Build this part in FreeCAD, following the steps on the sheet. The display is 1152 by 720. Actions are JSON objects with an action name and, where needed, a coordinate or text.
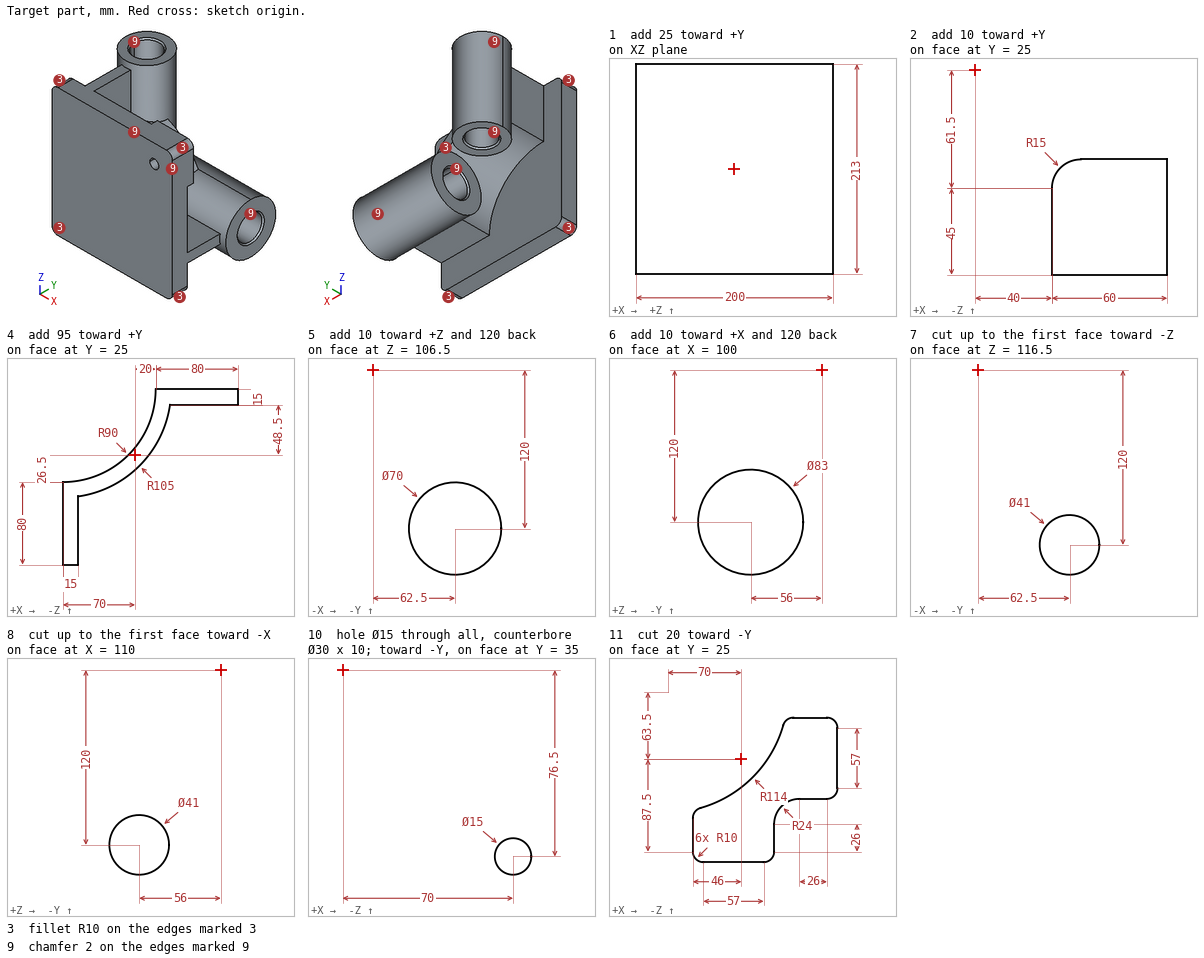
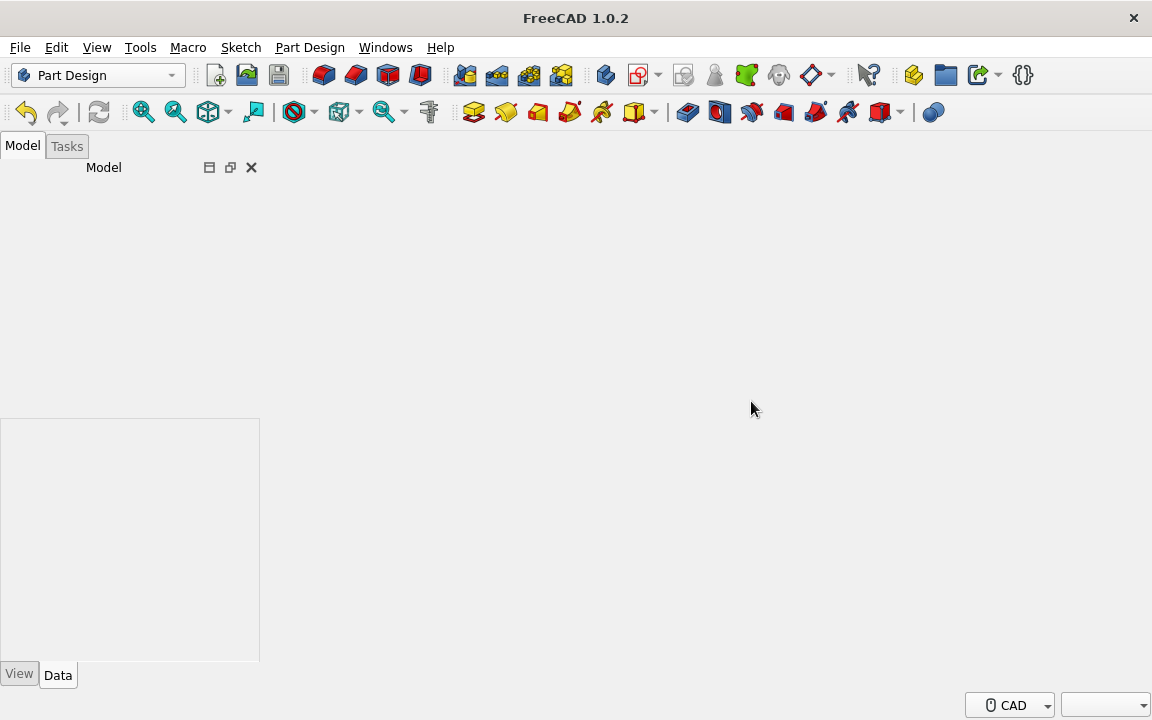
{"action": "left_click", "coordinate": [216, 76]}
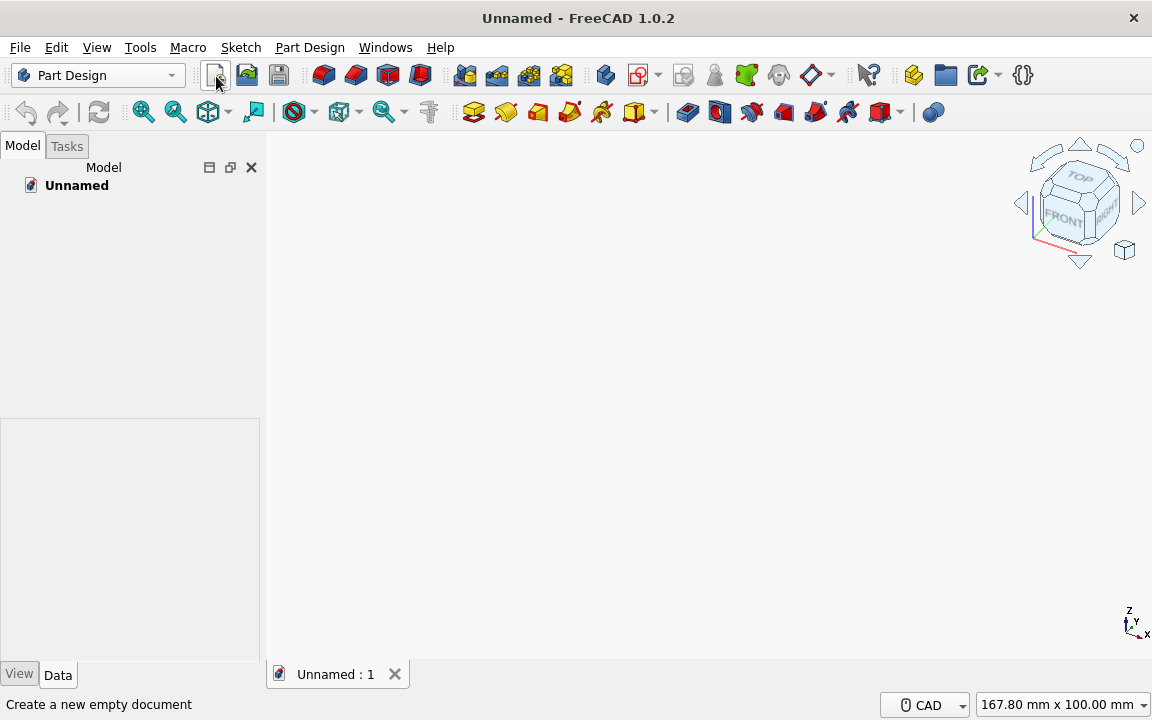
{"action": "left_click", "coordinate": [638, 76]}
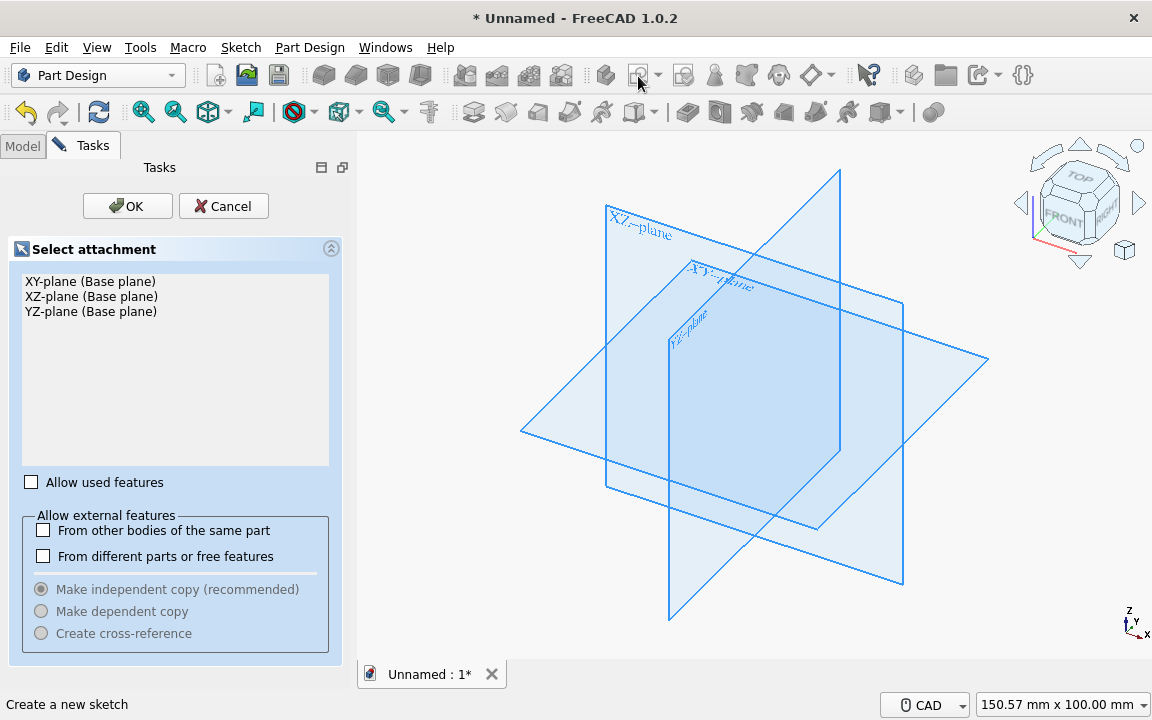
{"action": "left_click", "coordinate": [82, 296]}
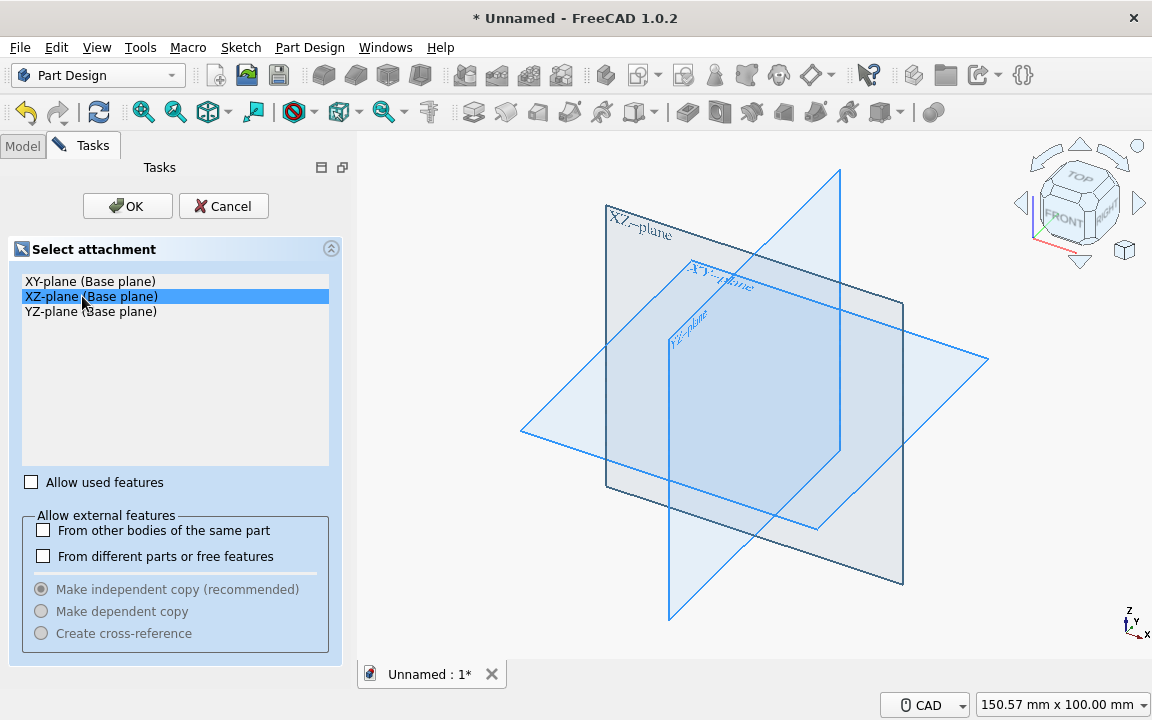
{"action": "left_click", "coordinate": [128, 206]}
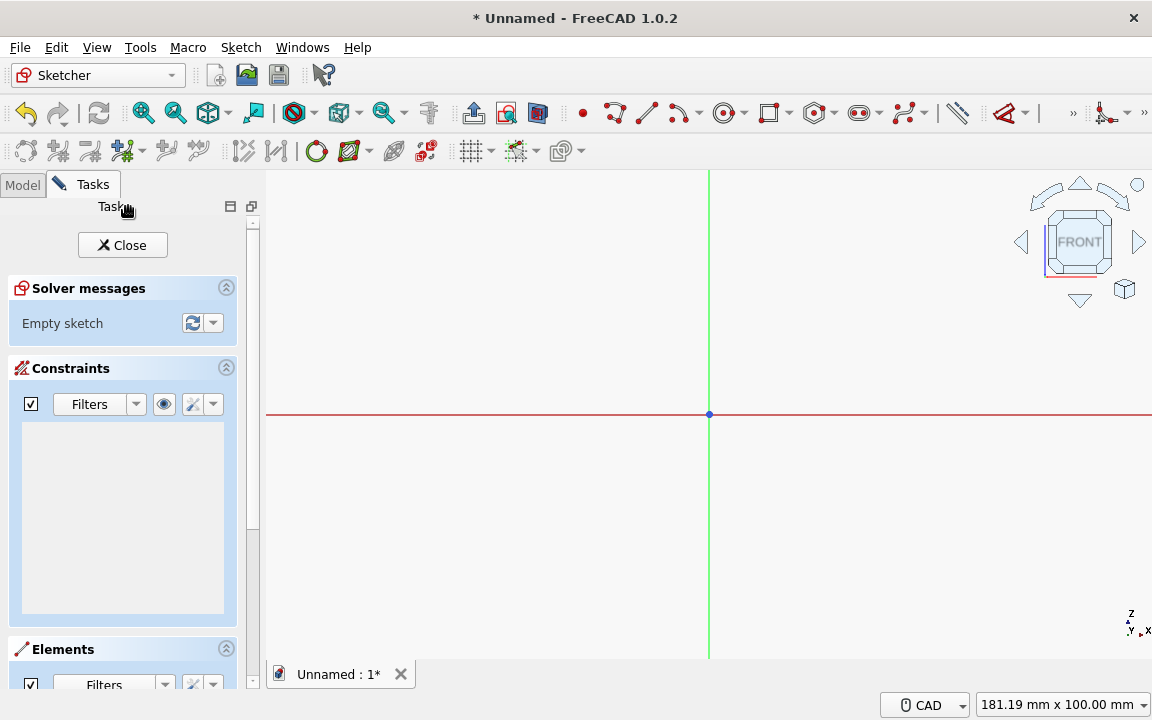
{"action": "scroll", "coordinate": [611, 414], "scroll_direction": "down", "scroll_amount": 6}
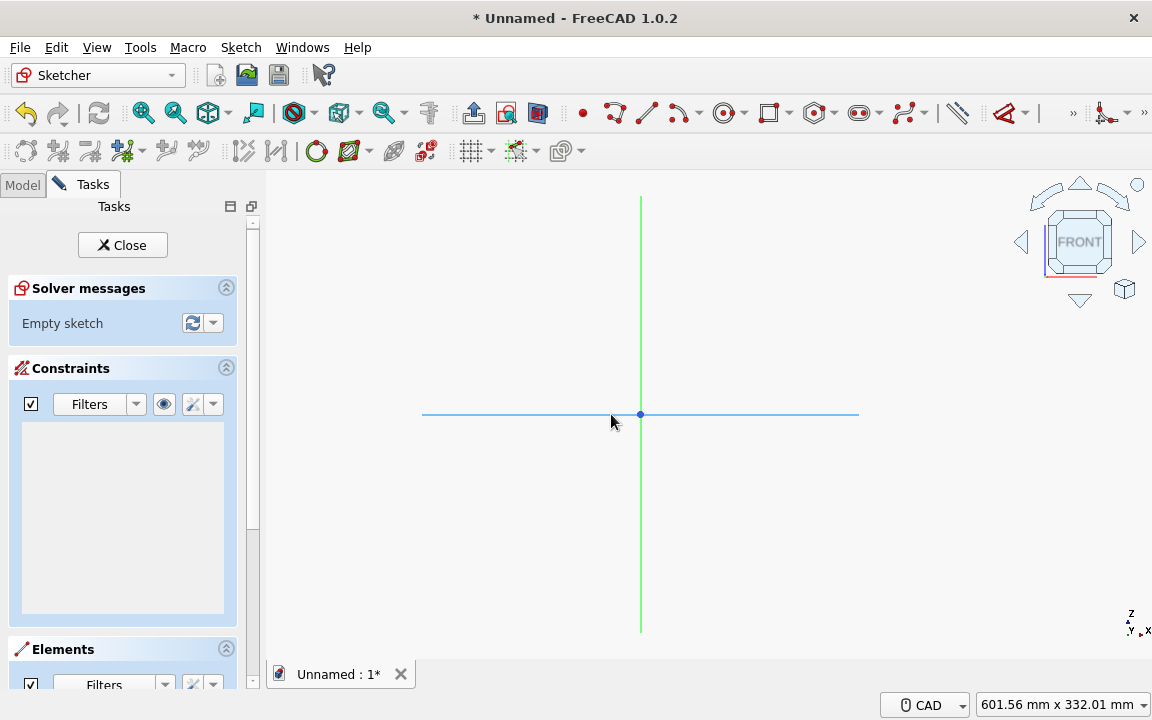
{"action": "left_click", "coordinate": [792, 114]}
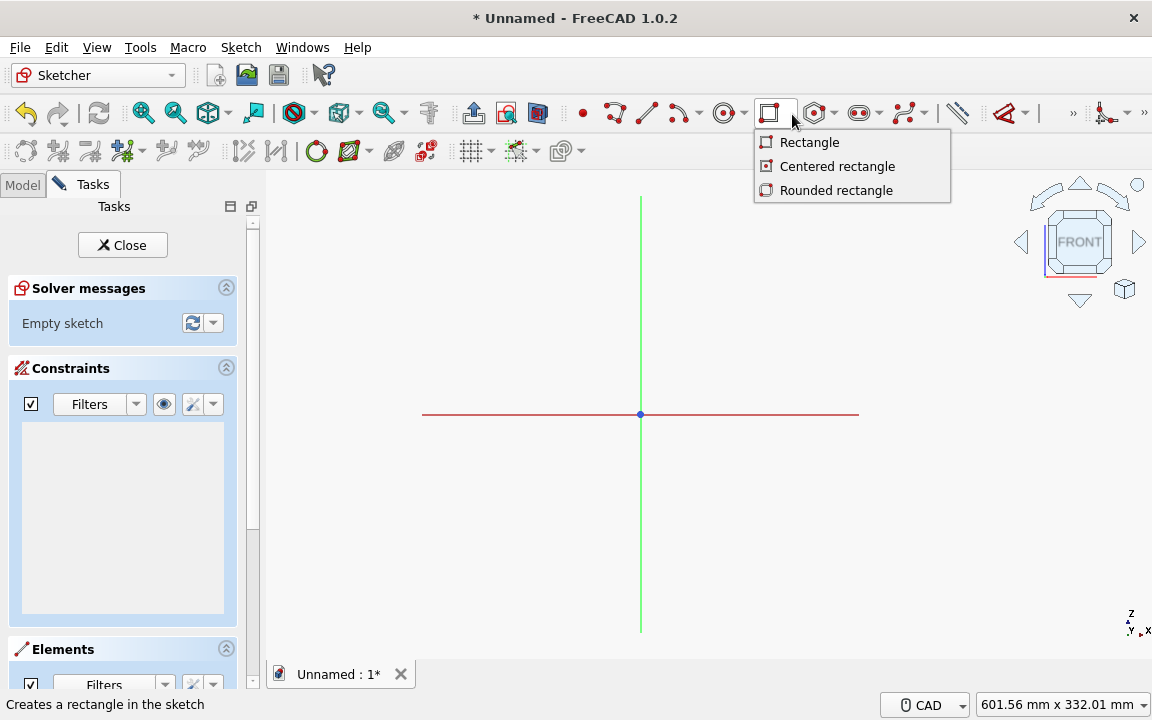
{"action": "left_click", "coordinate": [852, 166]}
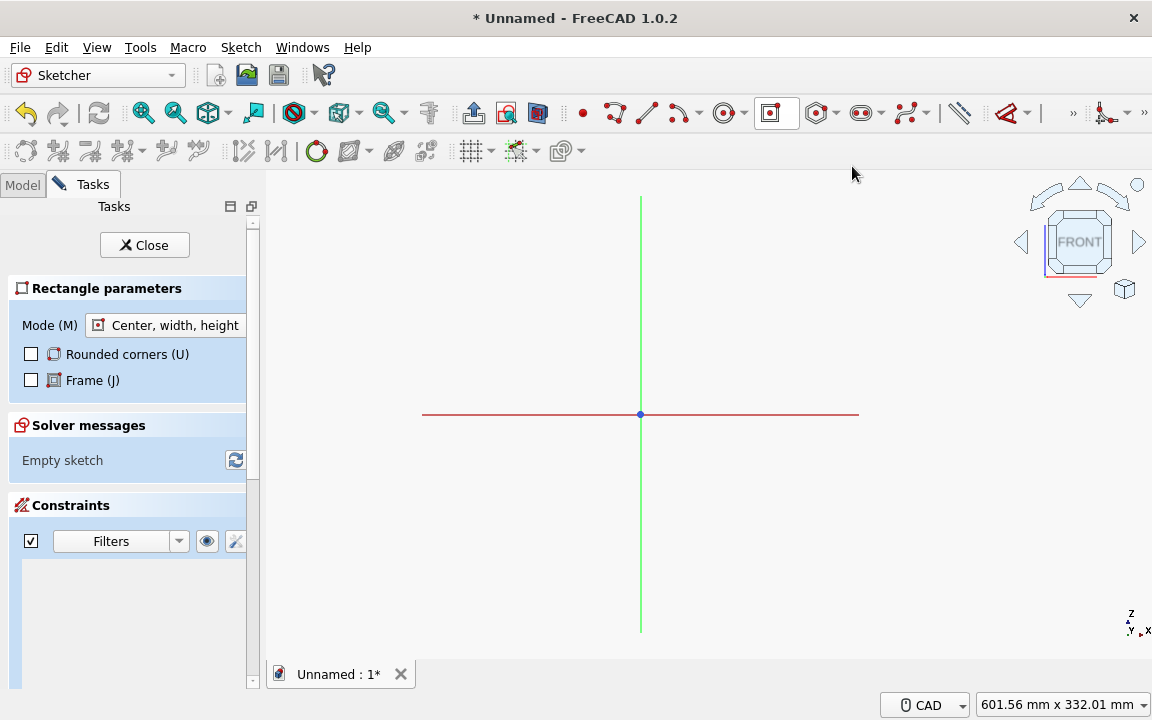
{"action": "left_click", "coordinate": [641, 414]}
{"action": "mouse_move", "coordinate": [788, 258]}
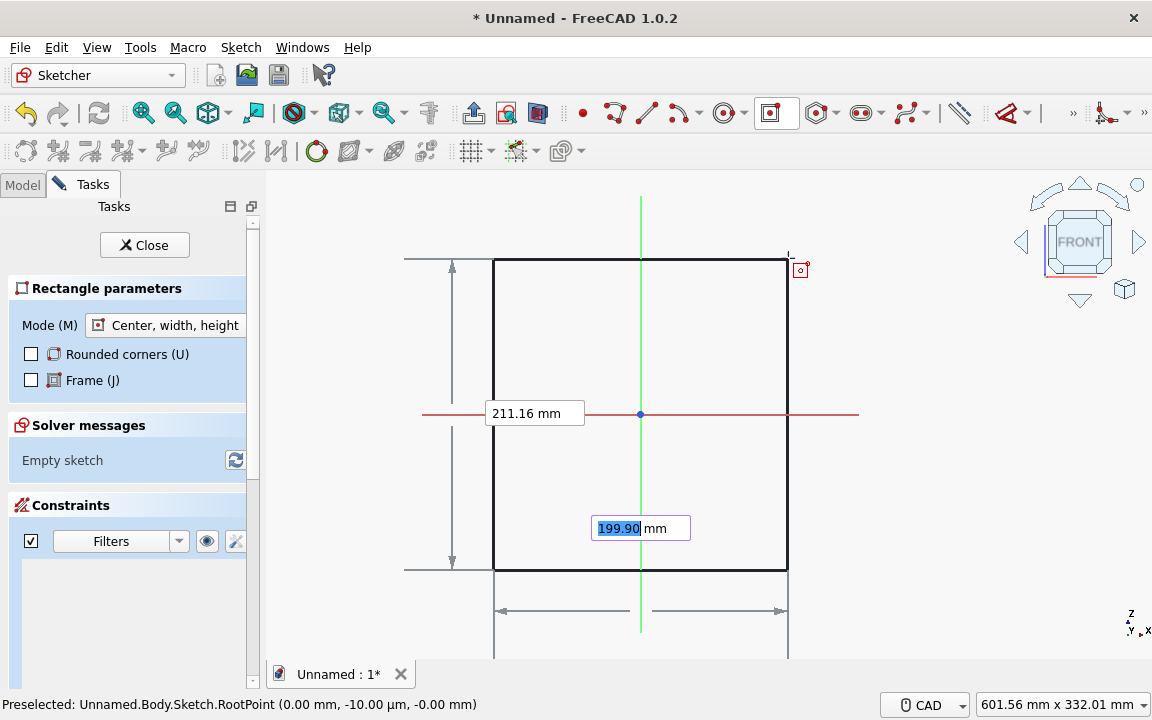
{"action": "type", "text": "200"}
{"action": "key", "text": "Tab"}
{"action": "type", "text": "213"}
{"action": "key", "text": "Return"}
{"action": "key", "text": "Escape"}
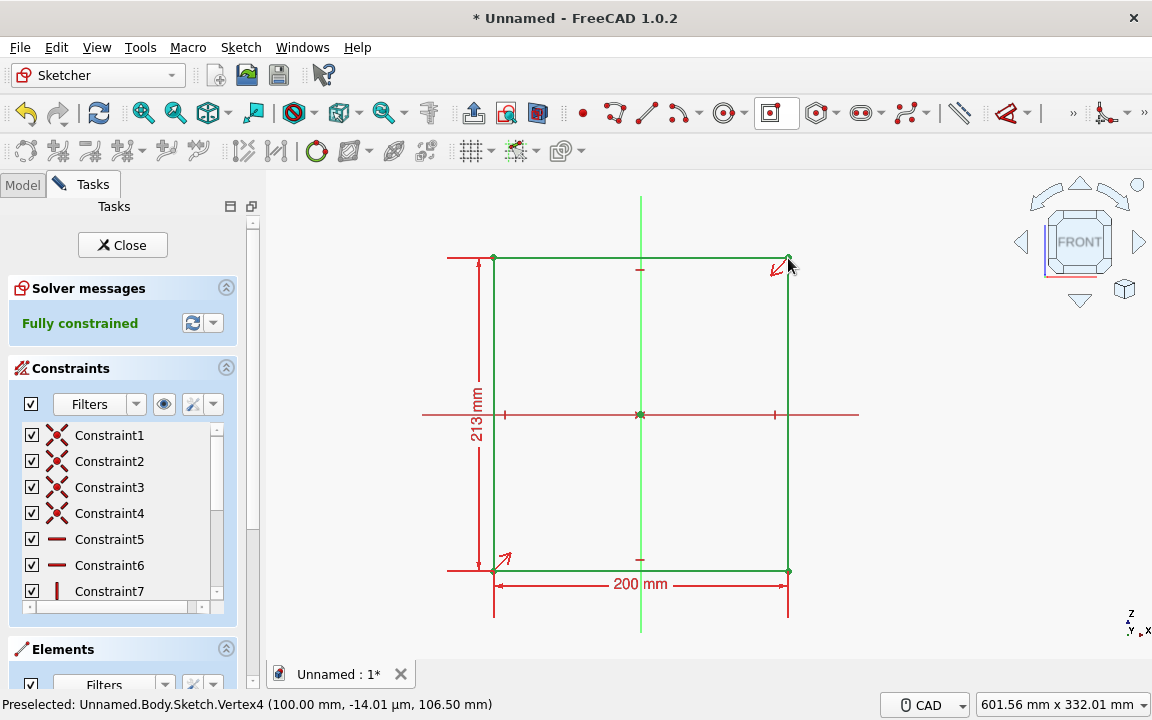
{"action": "left_click", "coordinate": [123, 245]}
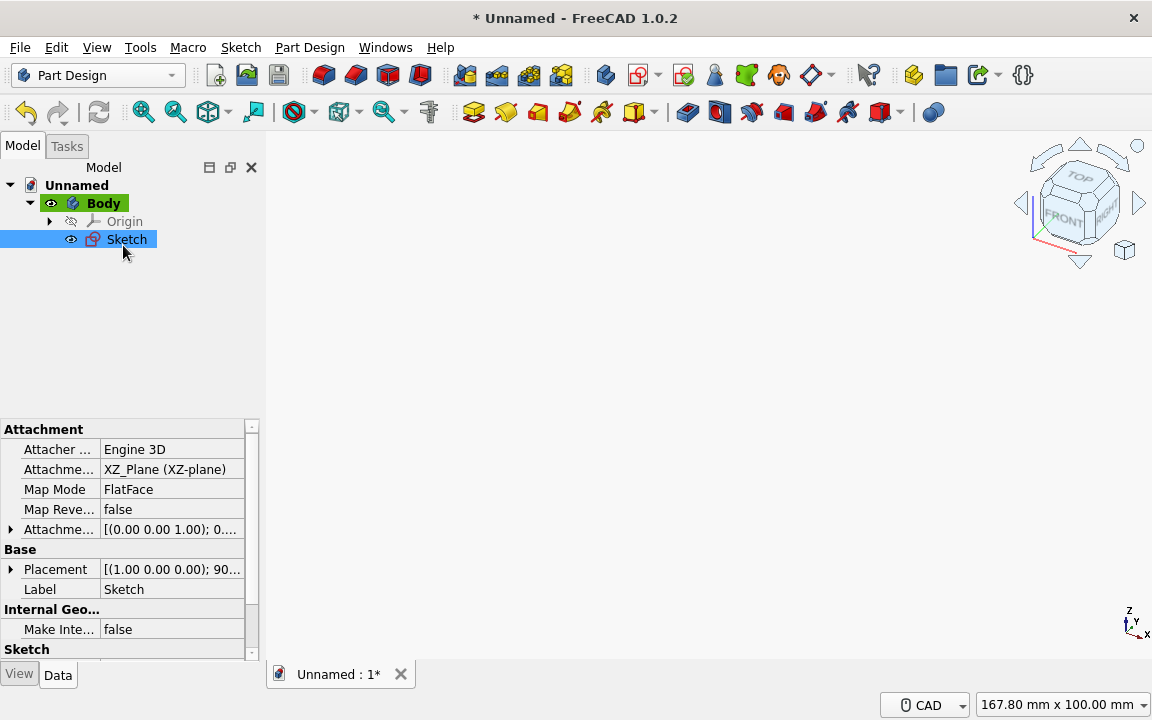
{"action": "left_click", "coordinate": [474, 112]}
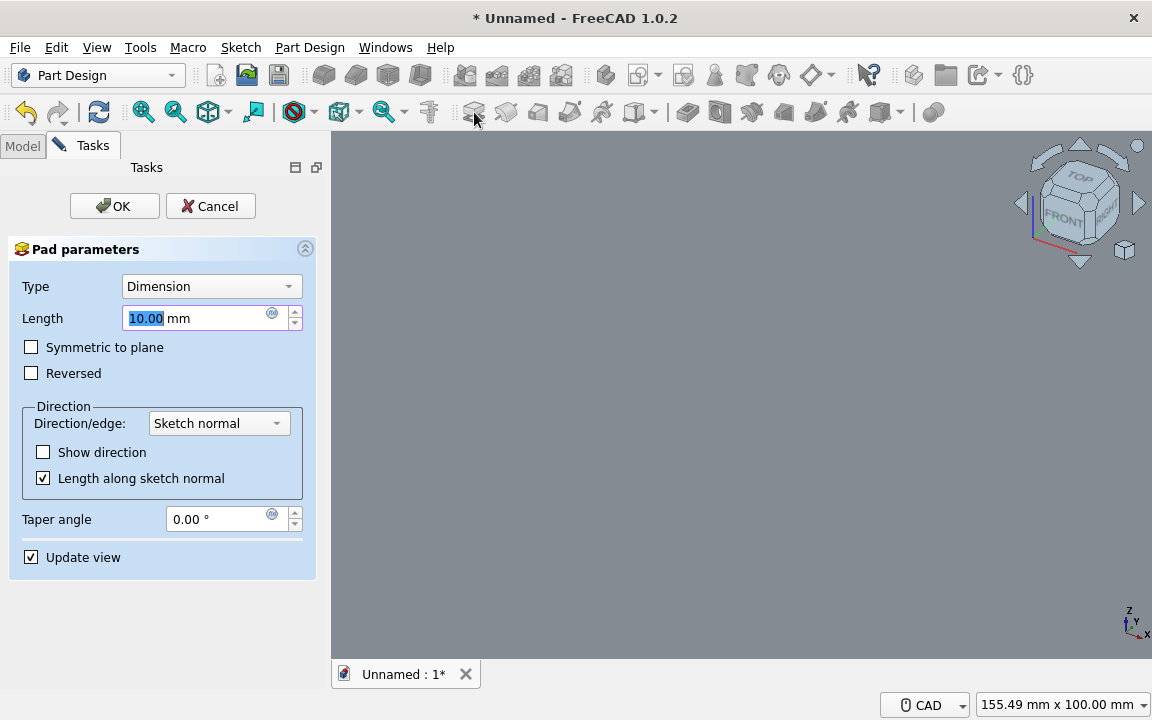
{"action": "type", "text": "25"}
{"action": "key", "text": "Tab"}